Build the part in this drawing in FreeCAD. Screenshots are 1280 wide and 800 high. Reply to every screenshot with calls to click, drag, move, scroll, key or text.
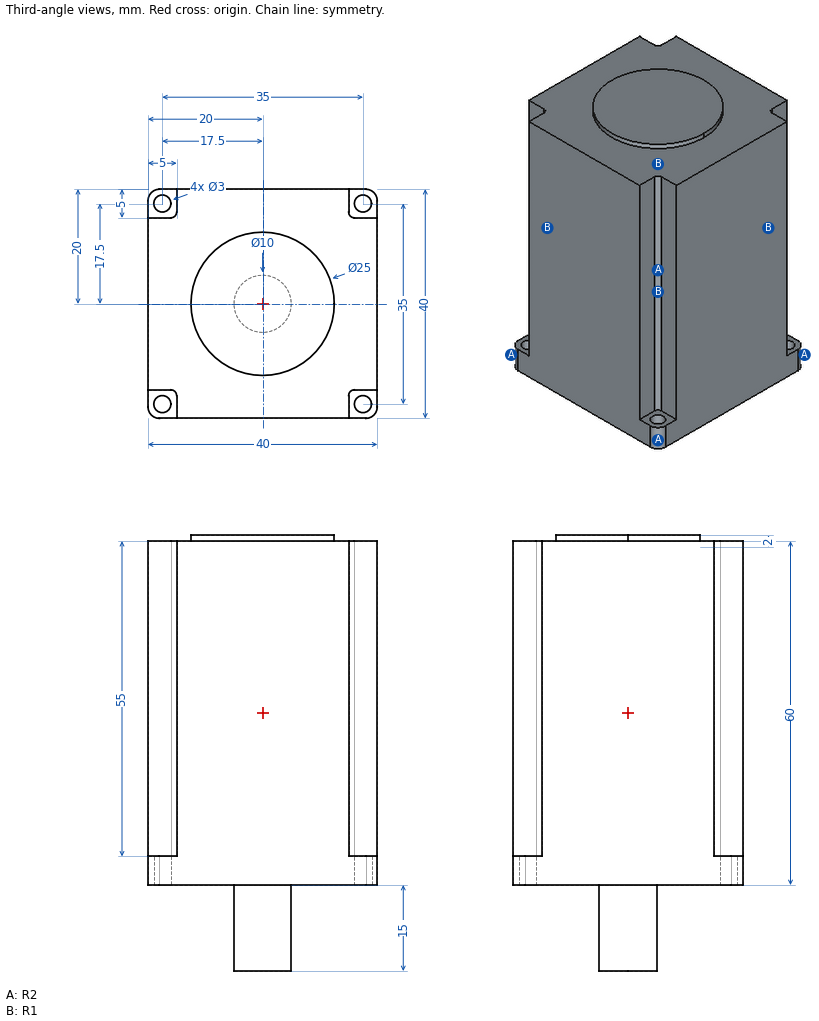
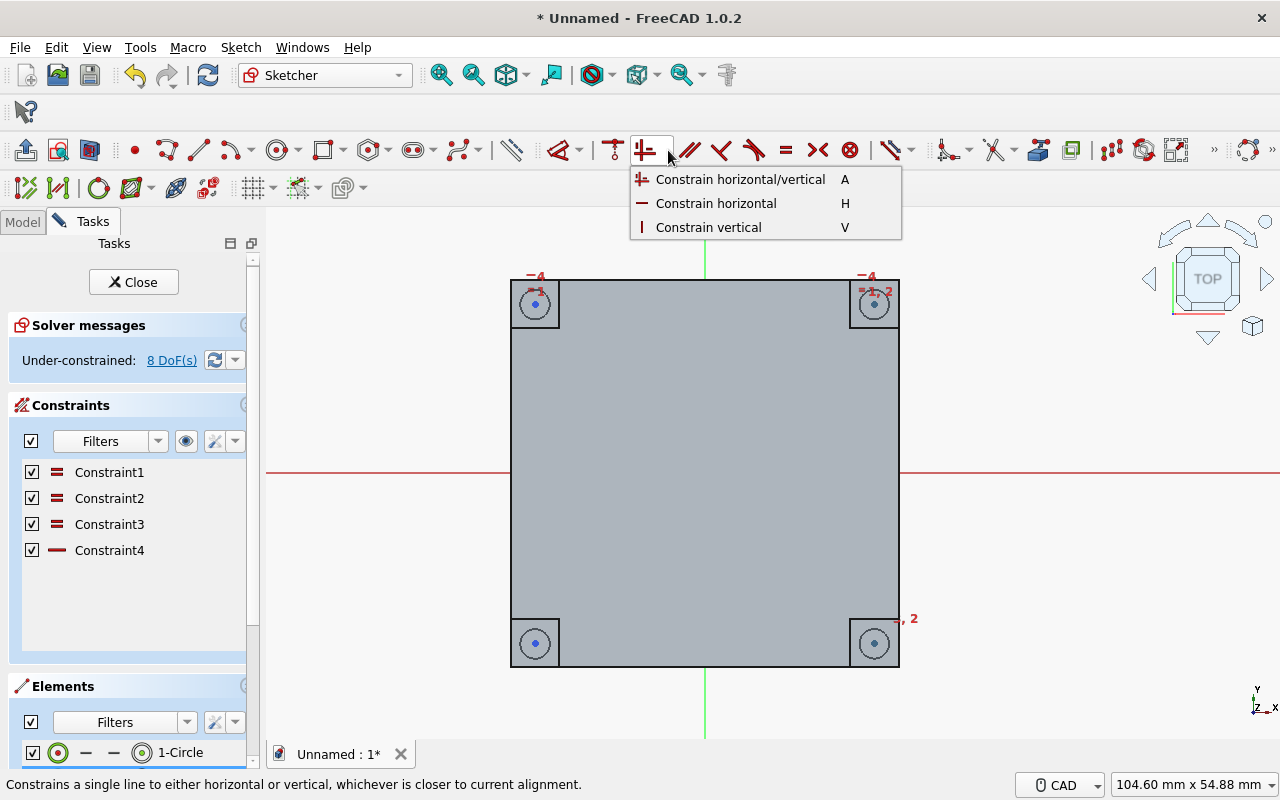
click(766, 227)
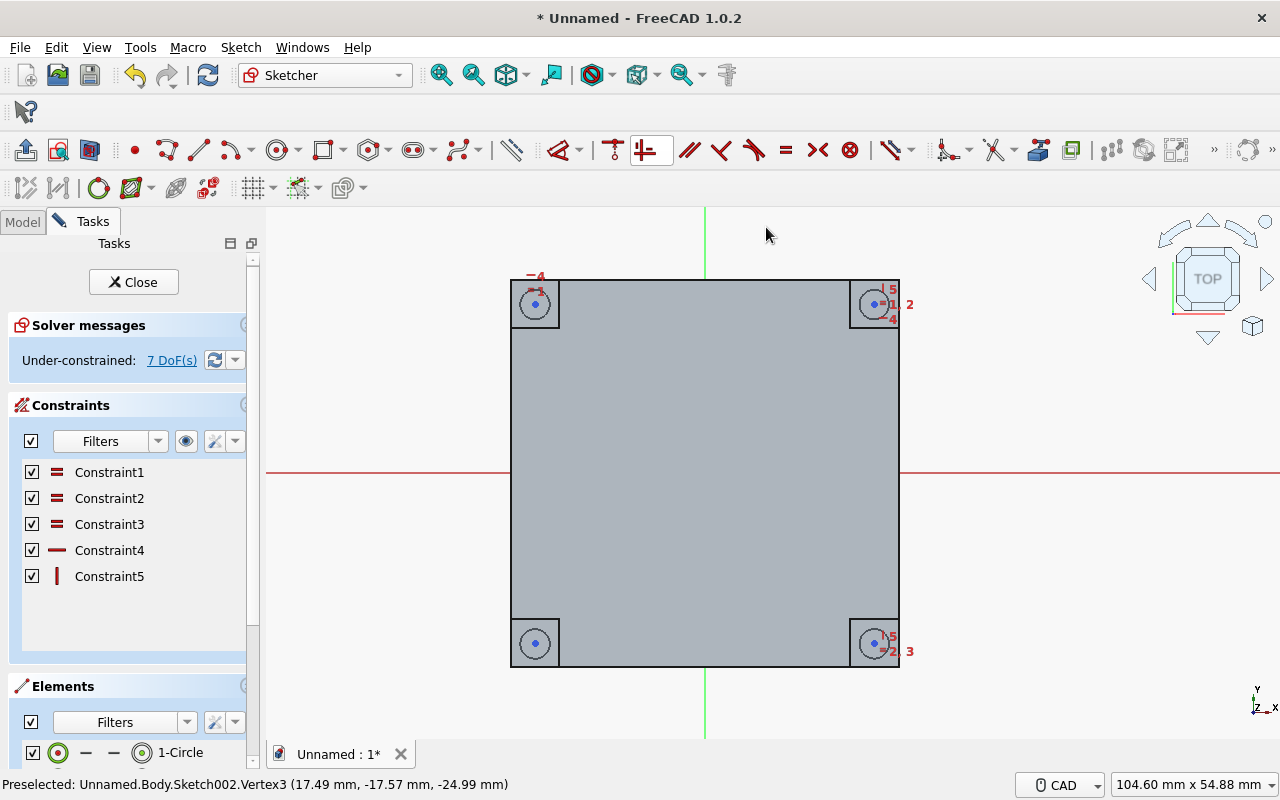
click(535, 305)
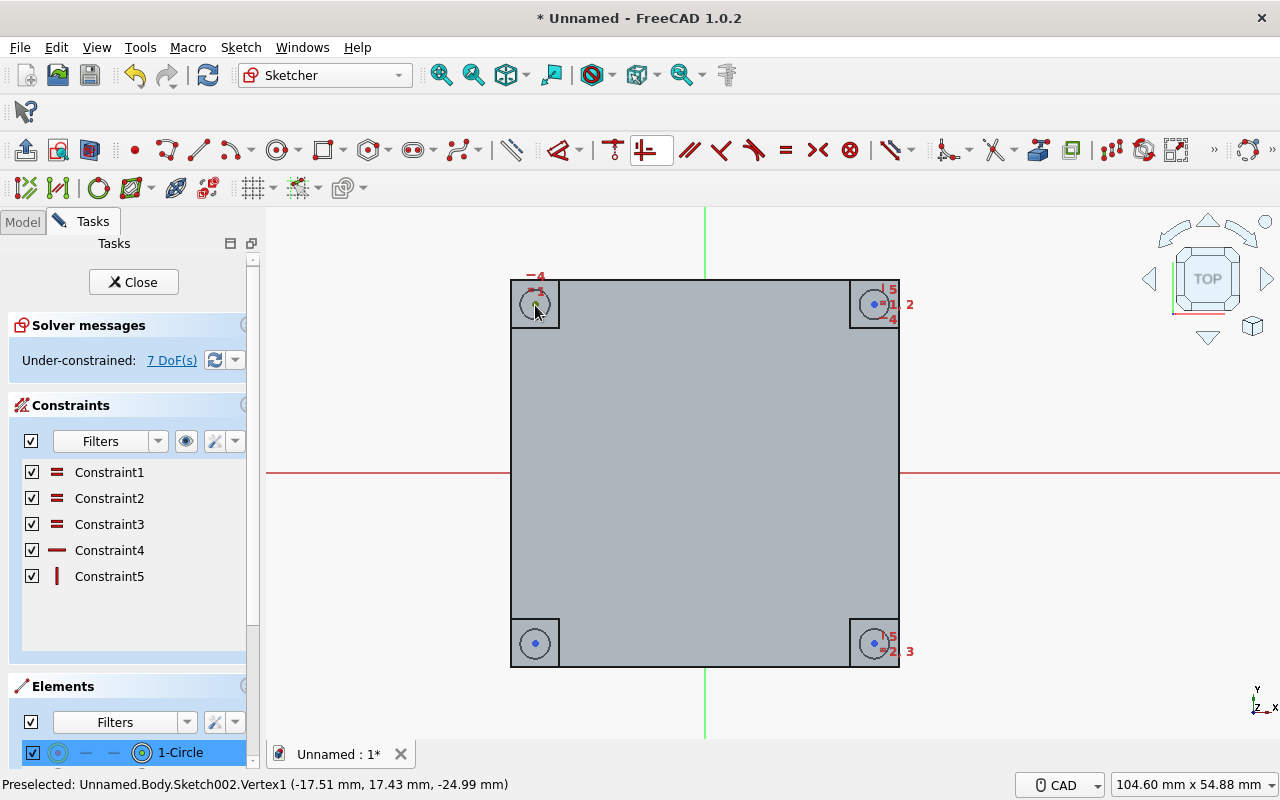
click(535, 644)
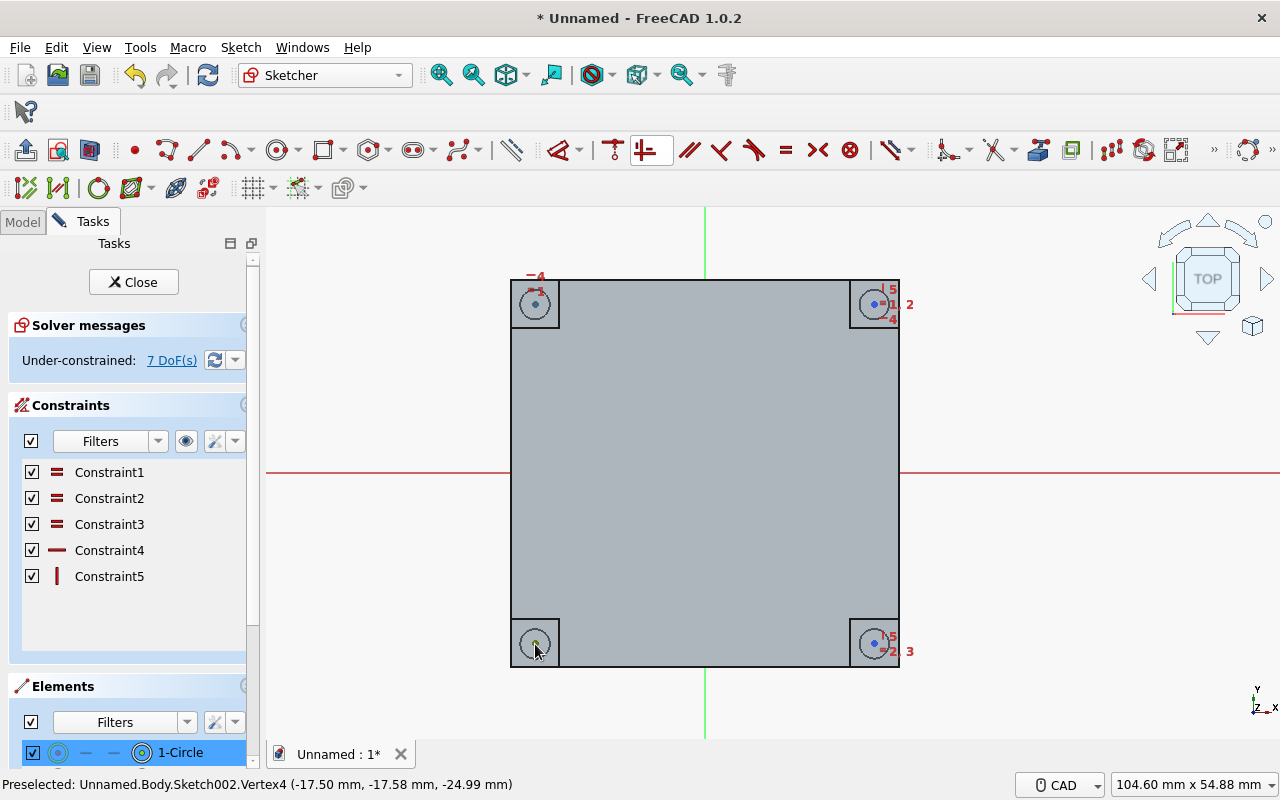
key(v)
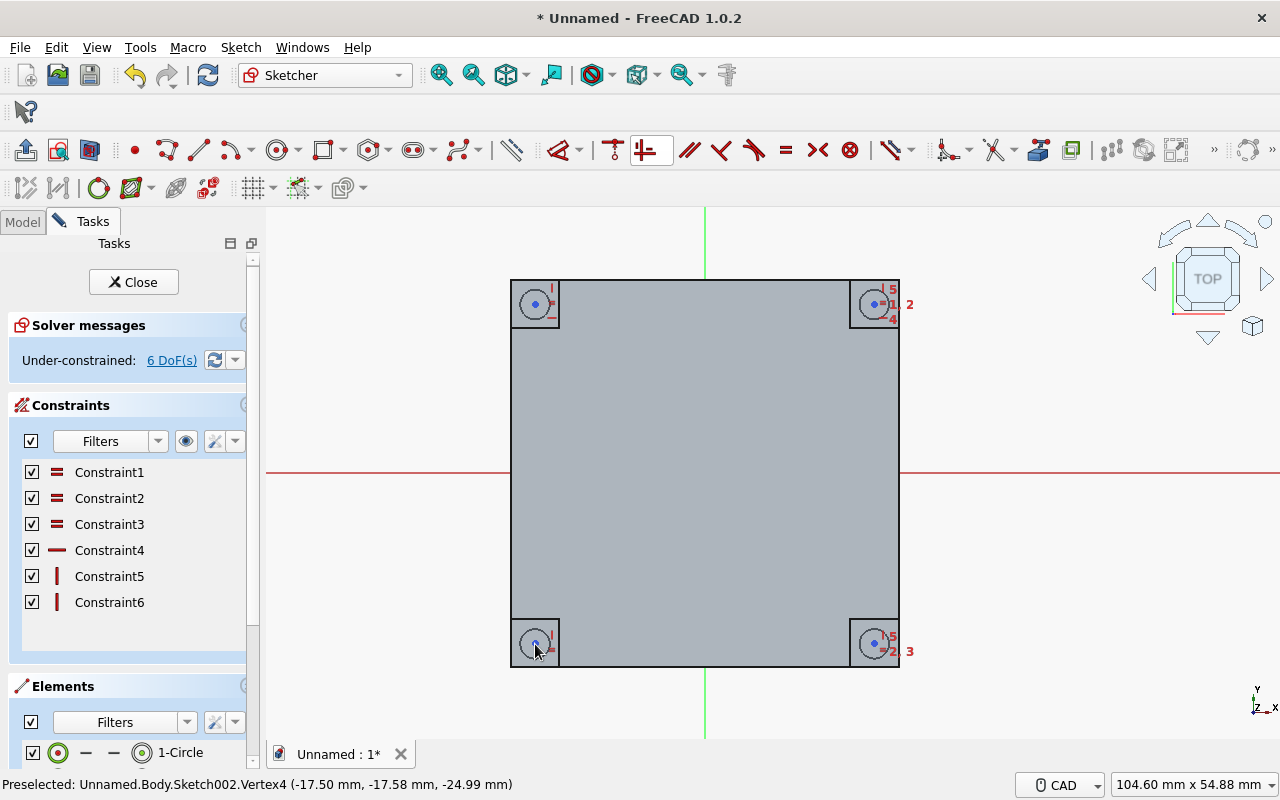
click(874, 644)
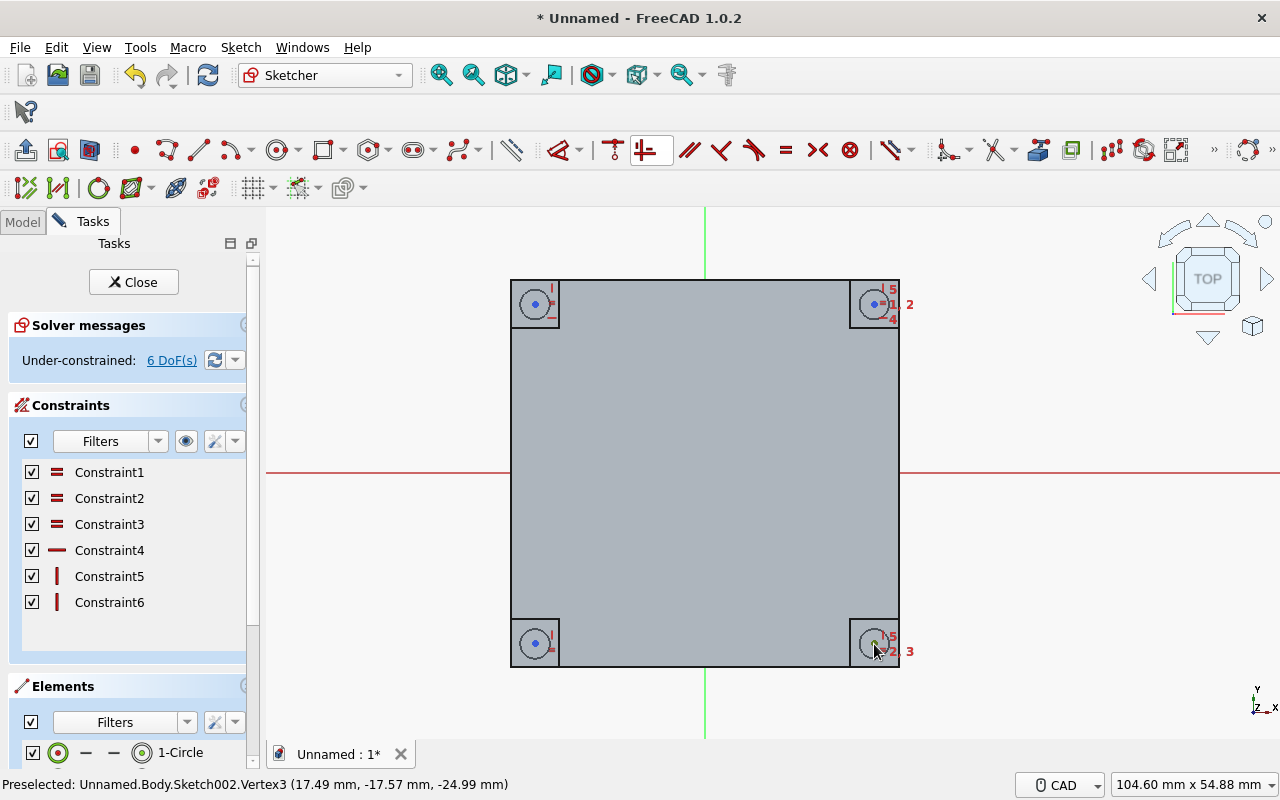
click(535, 644)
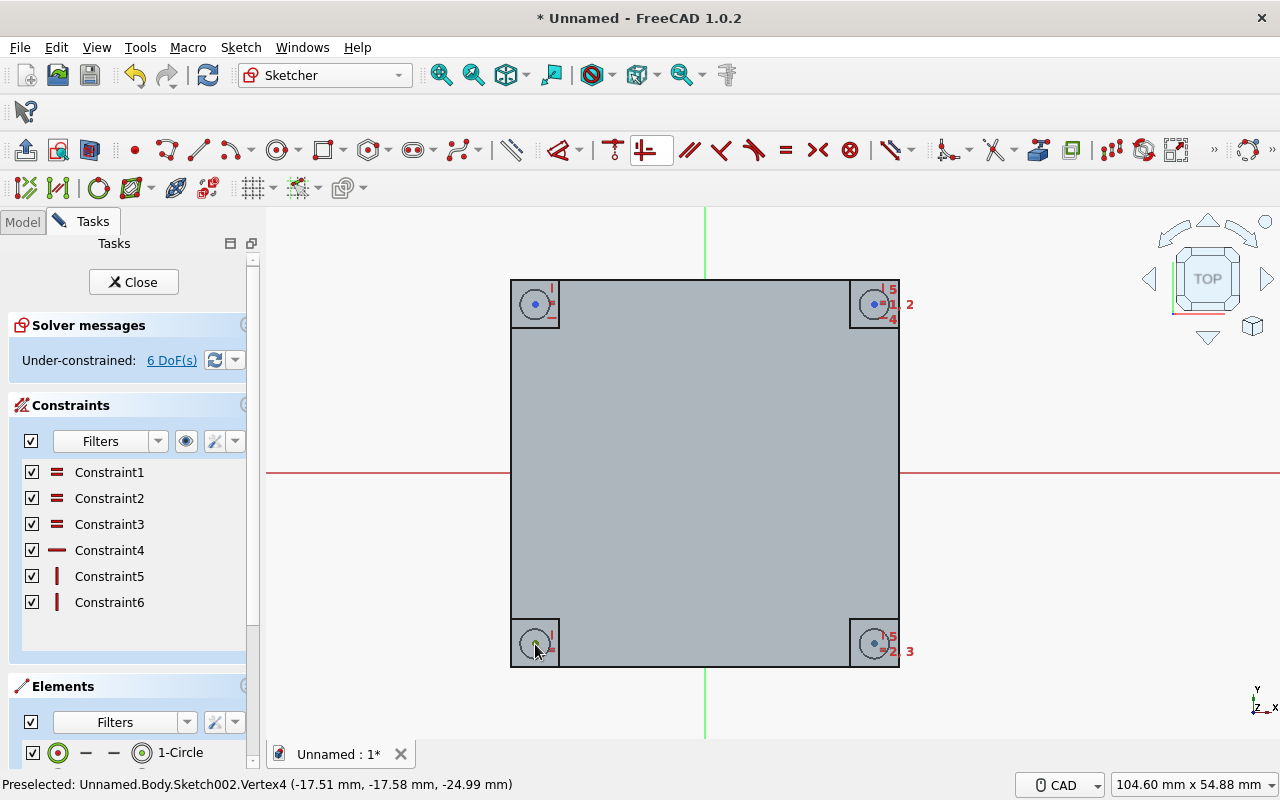
click(668, 150)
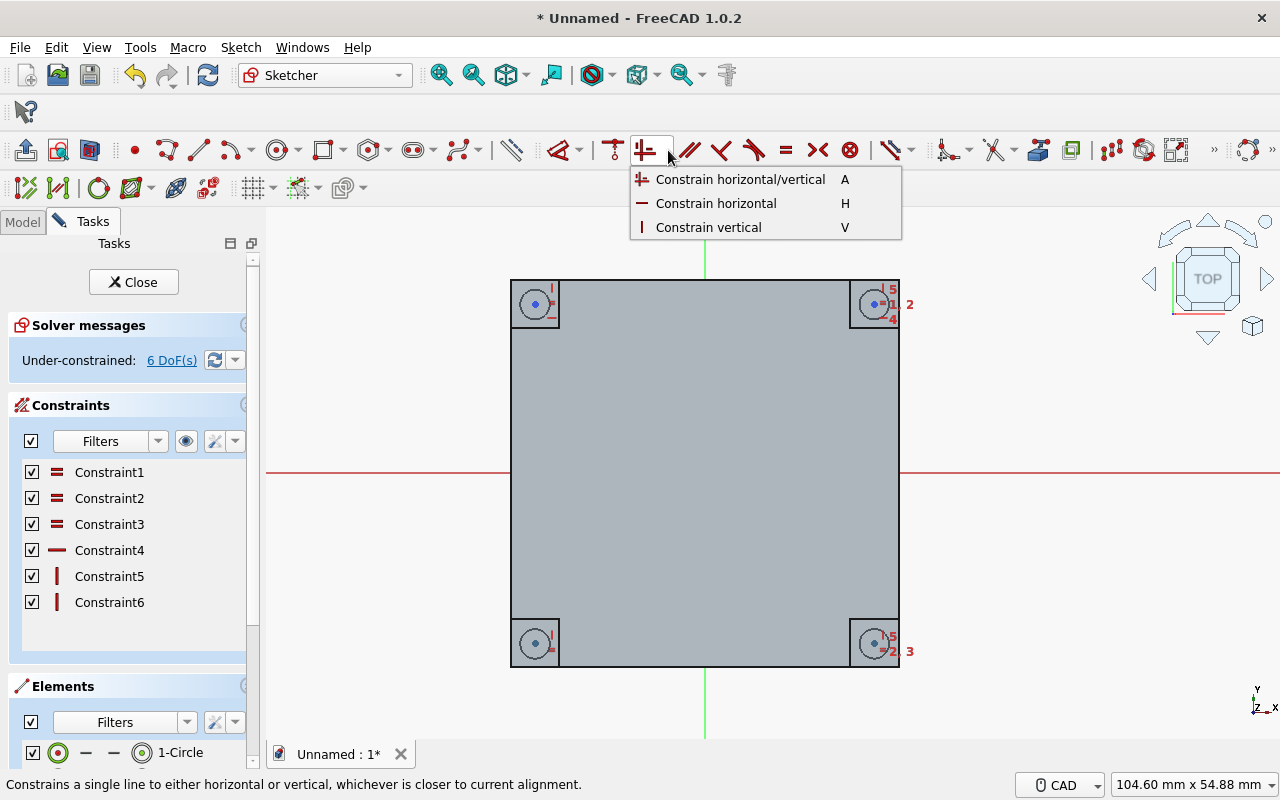
click(766, 203)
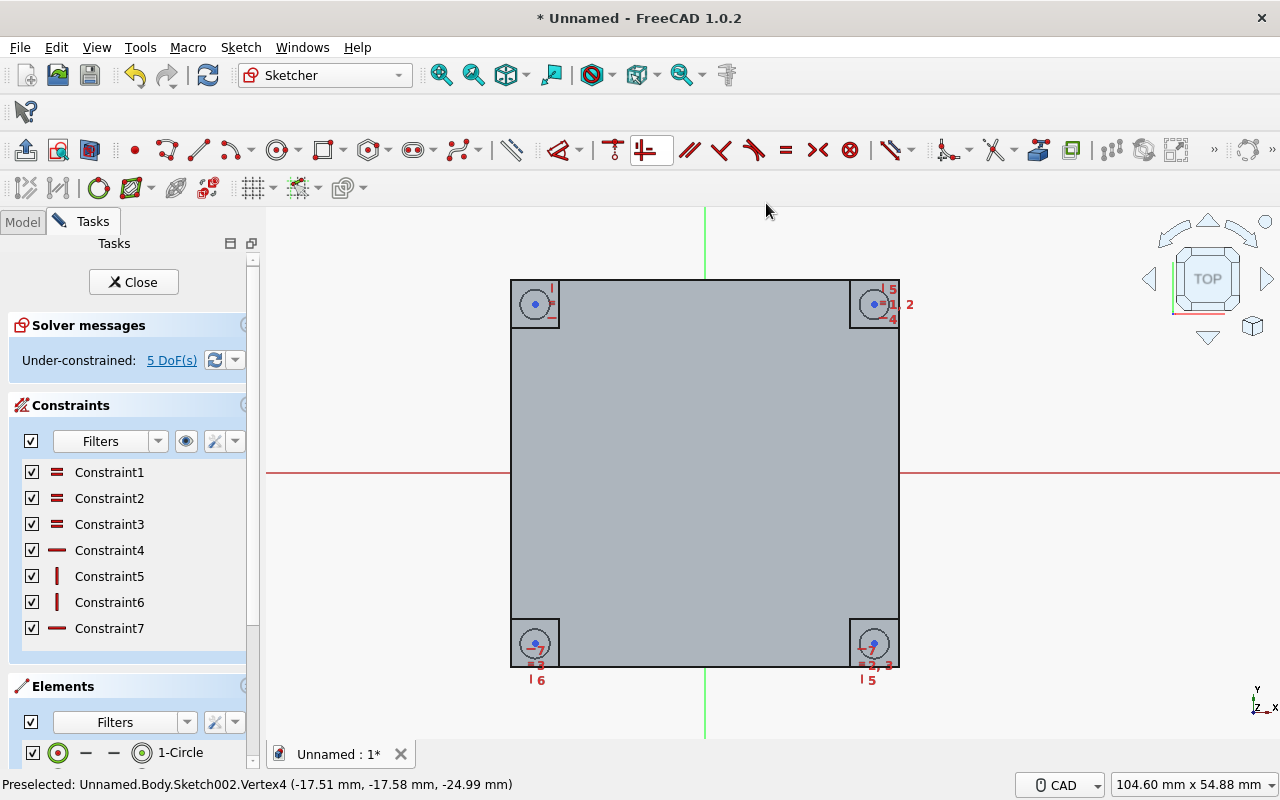
click(558, 150)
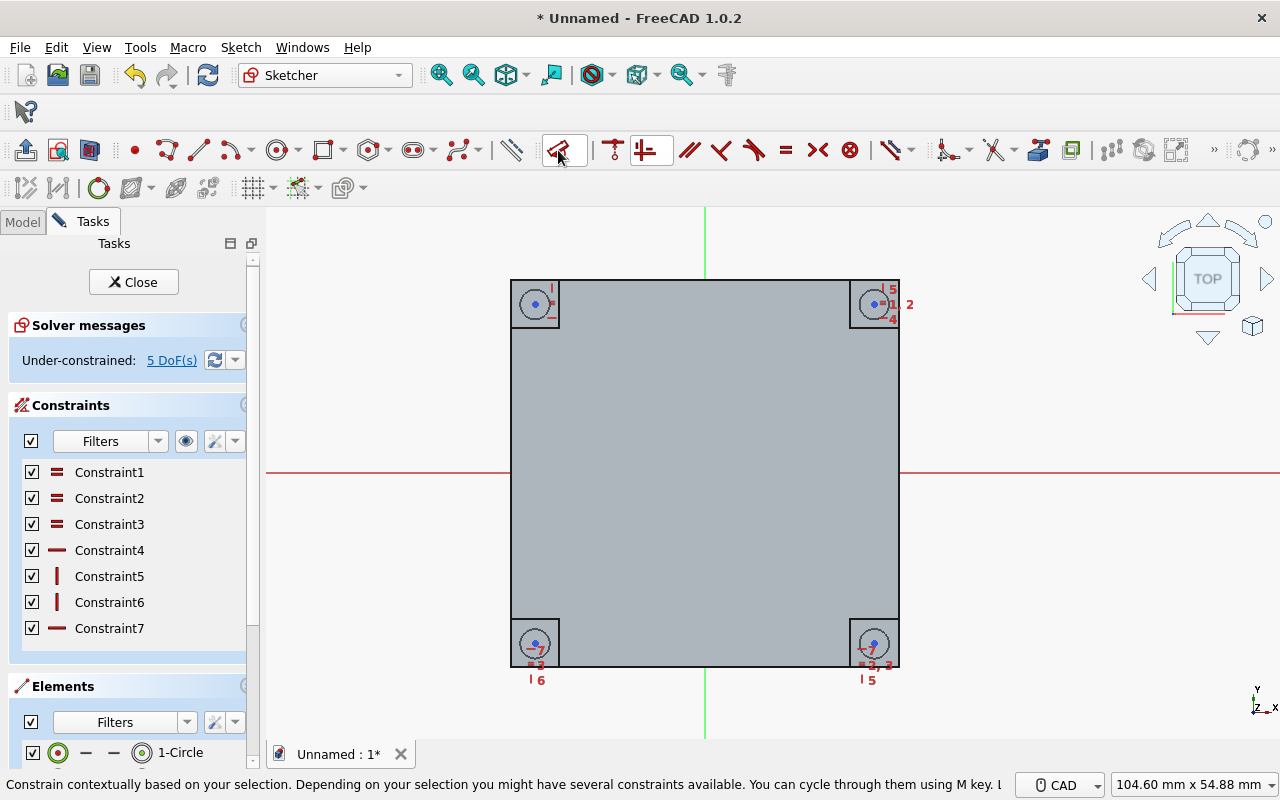
scroll(545, 294, up, 2)